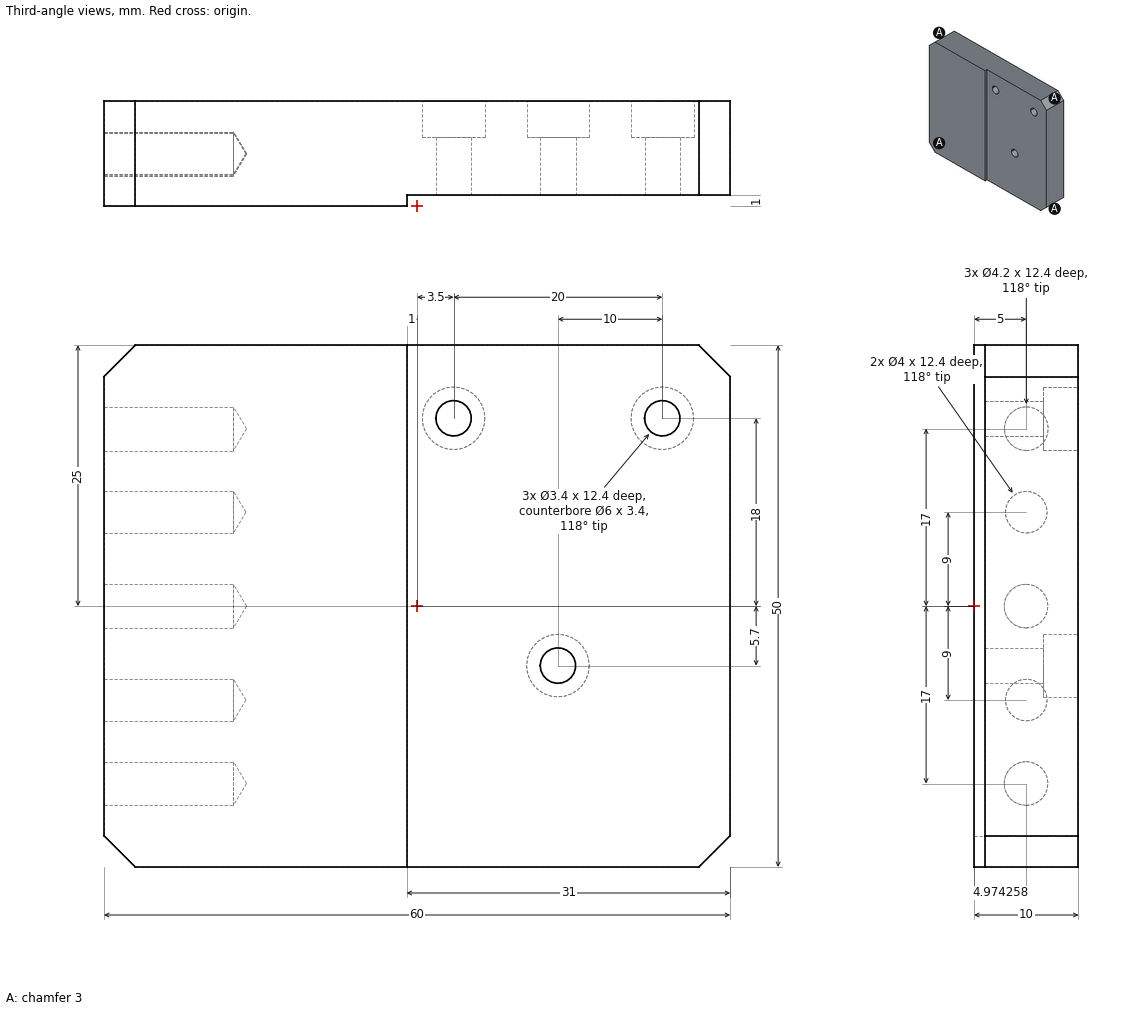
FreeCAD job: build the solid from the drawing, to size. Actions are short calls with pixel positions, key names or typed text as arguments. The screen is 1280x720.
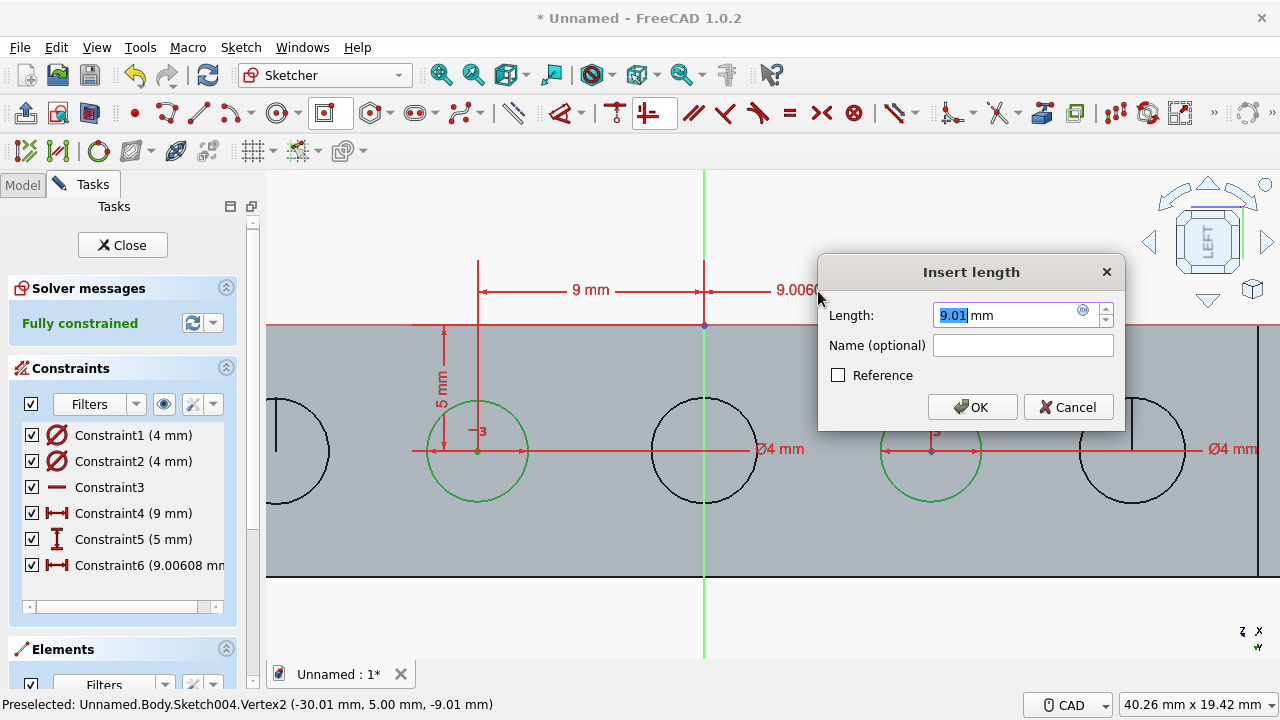
text(9)
key(Return)
key(Escape)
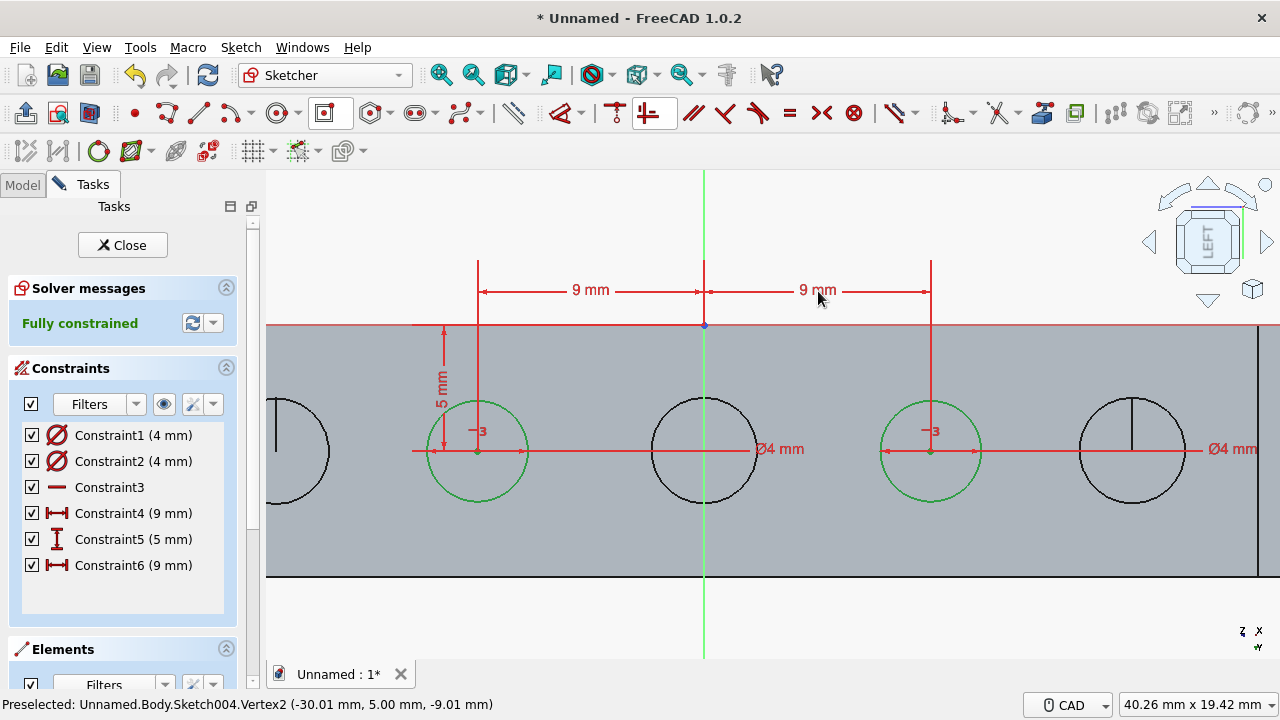
click(123, 245)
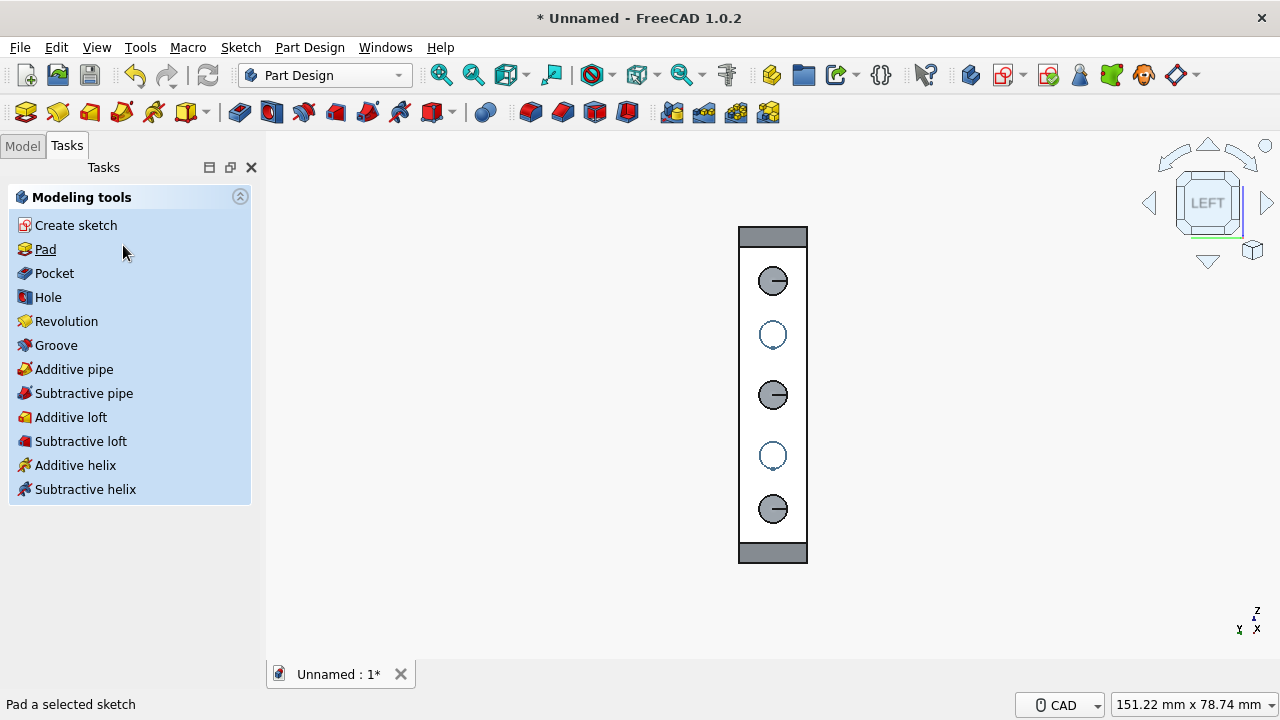
click(272, 112)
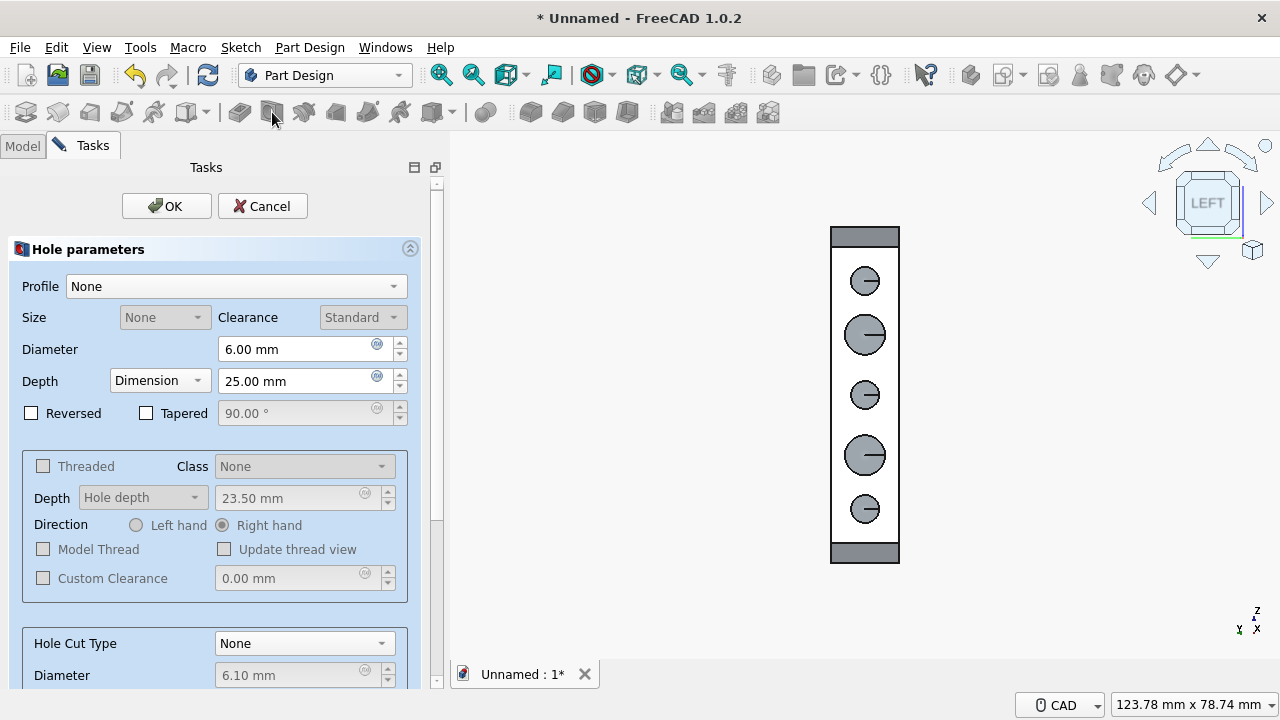
triple_click(305, 349)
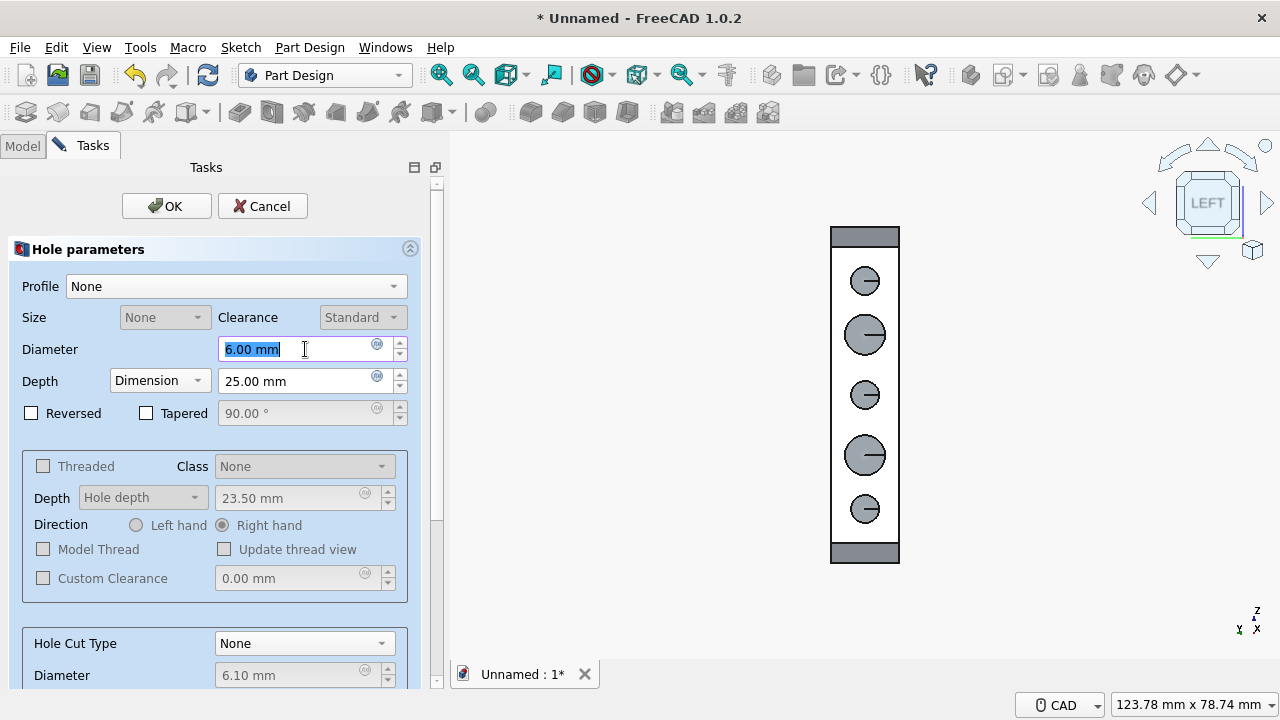
text(4)
key(Tab)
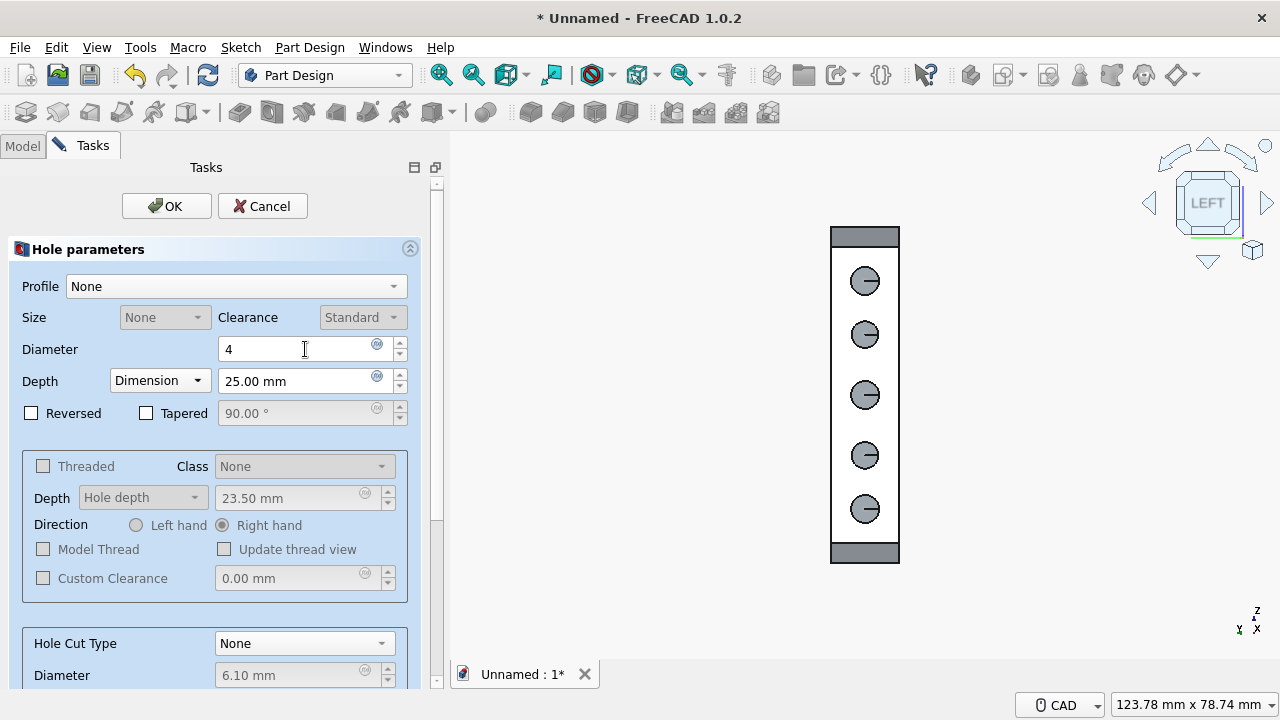
triple_click(305, 381)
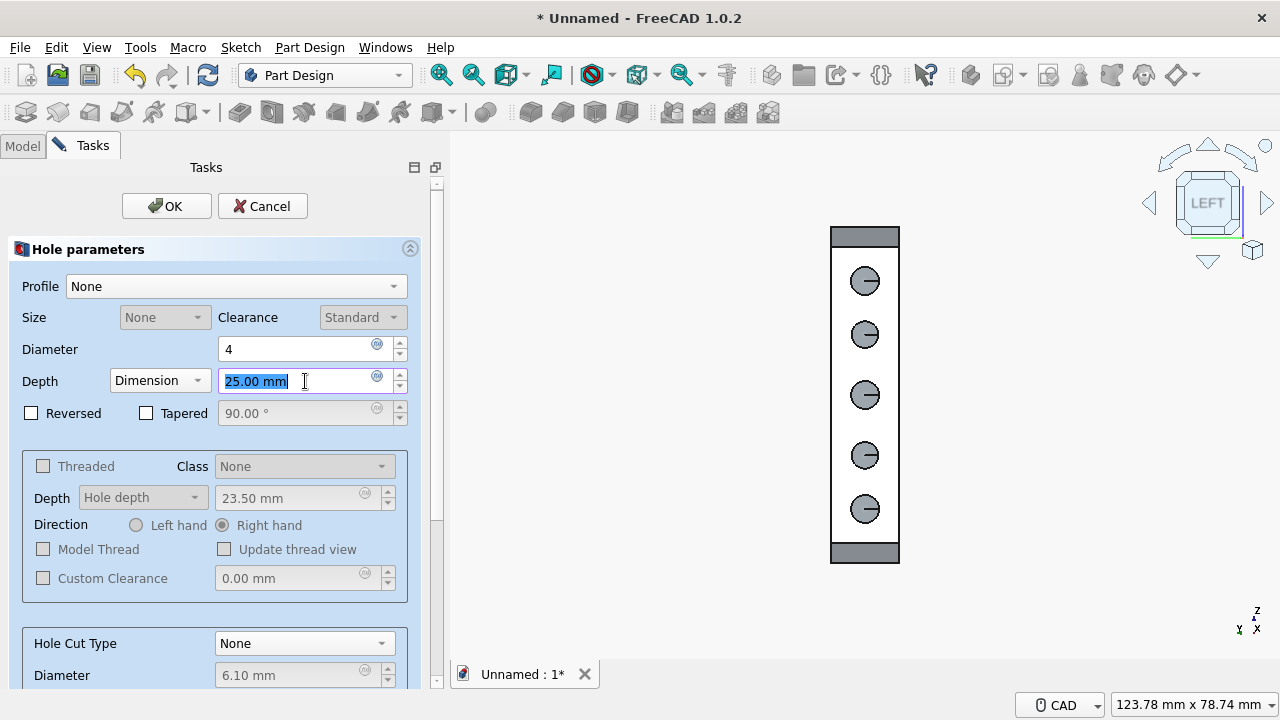
text(12.4)
key(Tab)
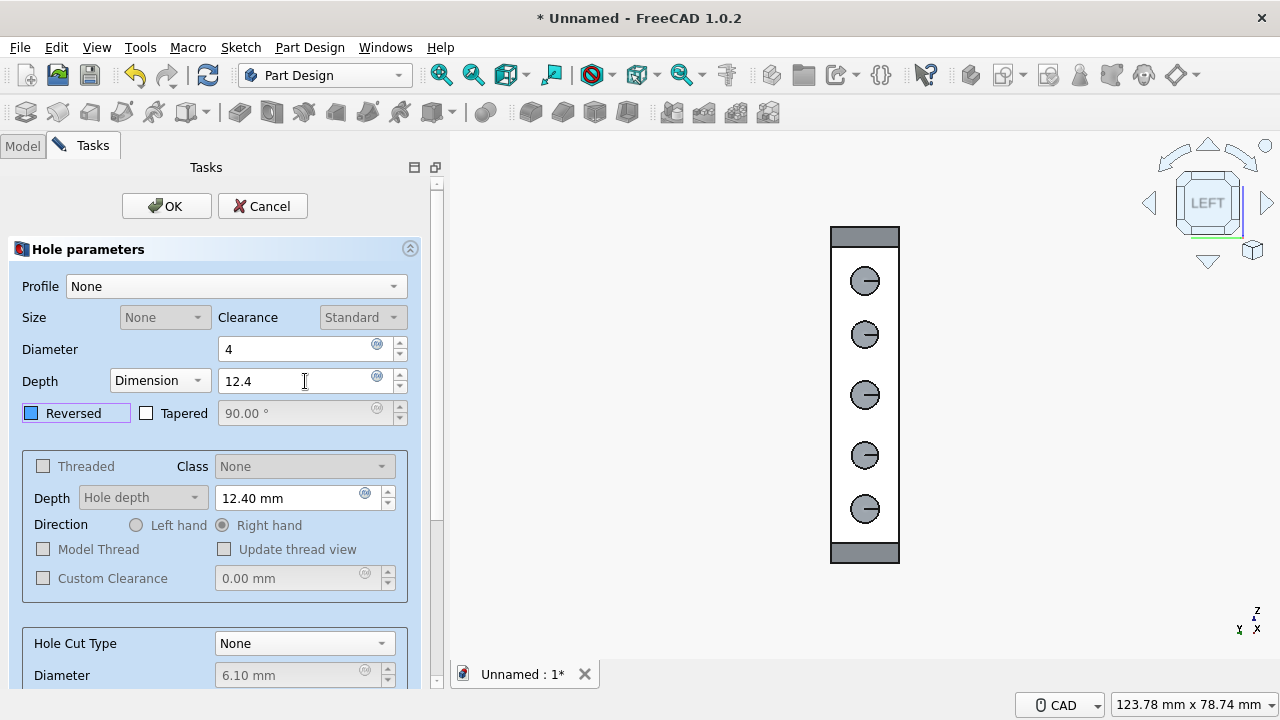
click(167, 206)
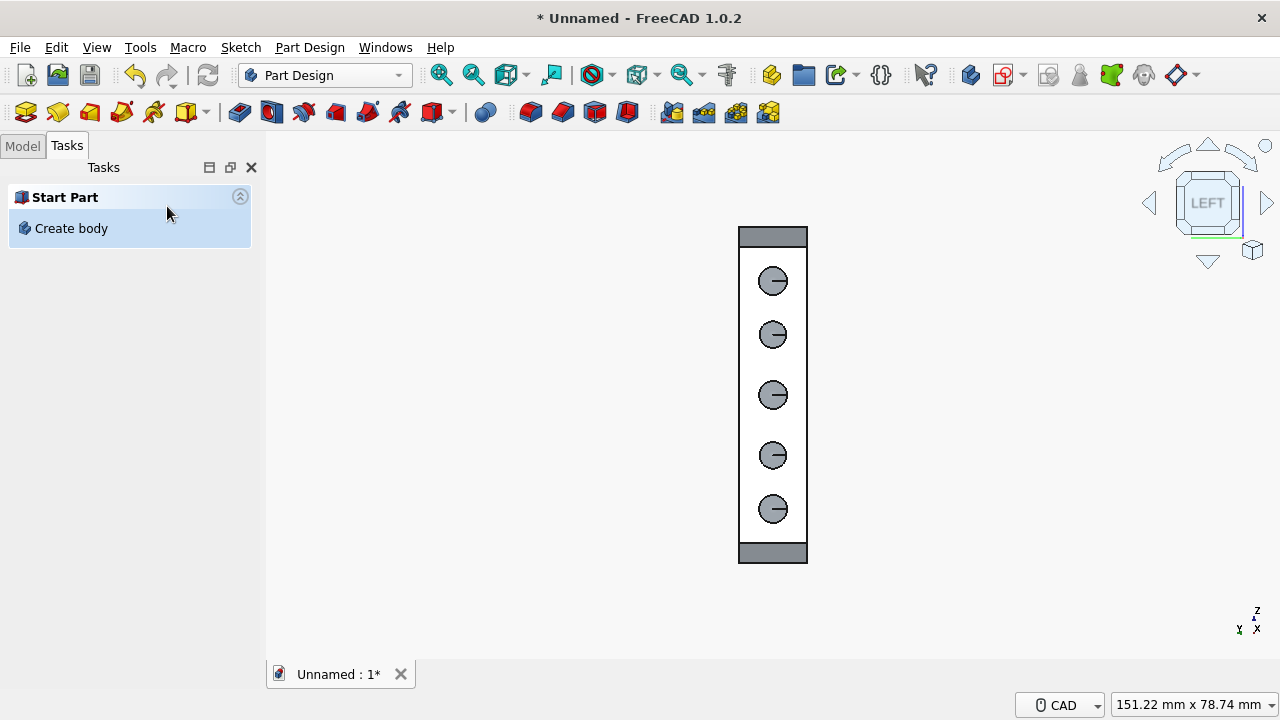
key(0)